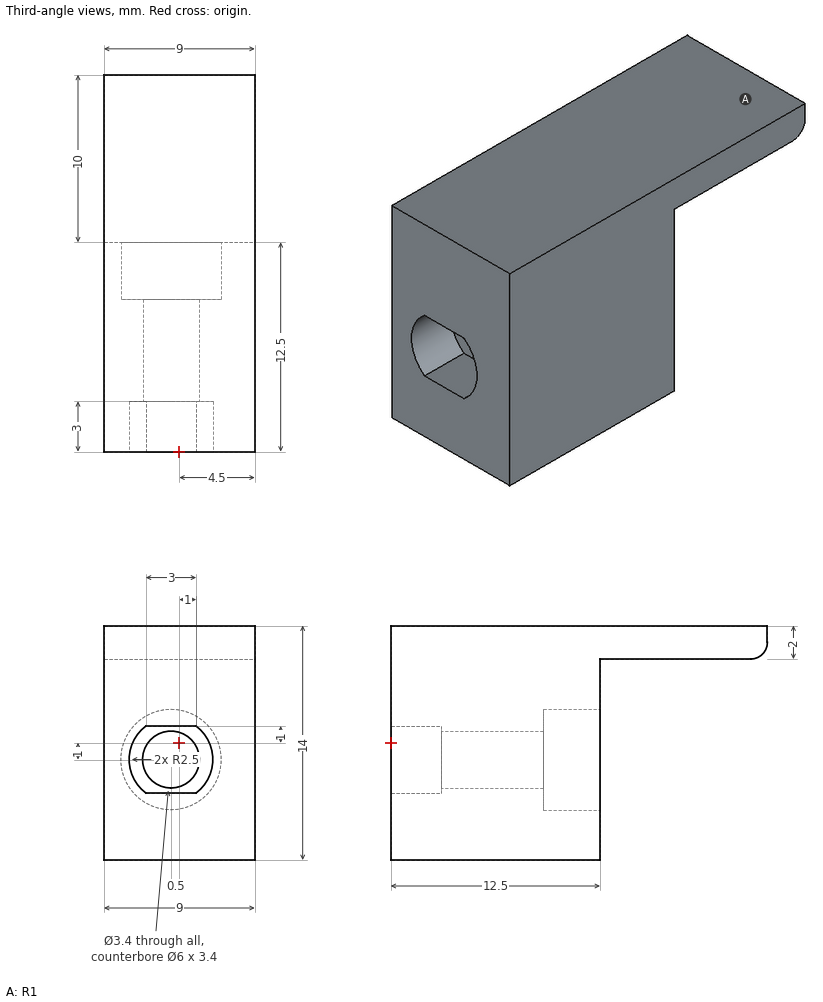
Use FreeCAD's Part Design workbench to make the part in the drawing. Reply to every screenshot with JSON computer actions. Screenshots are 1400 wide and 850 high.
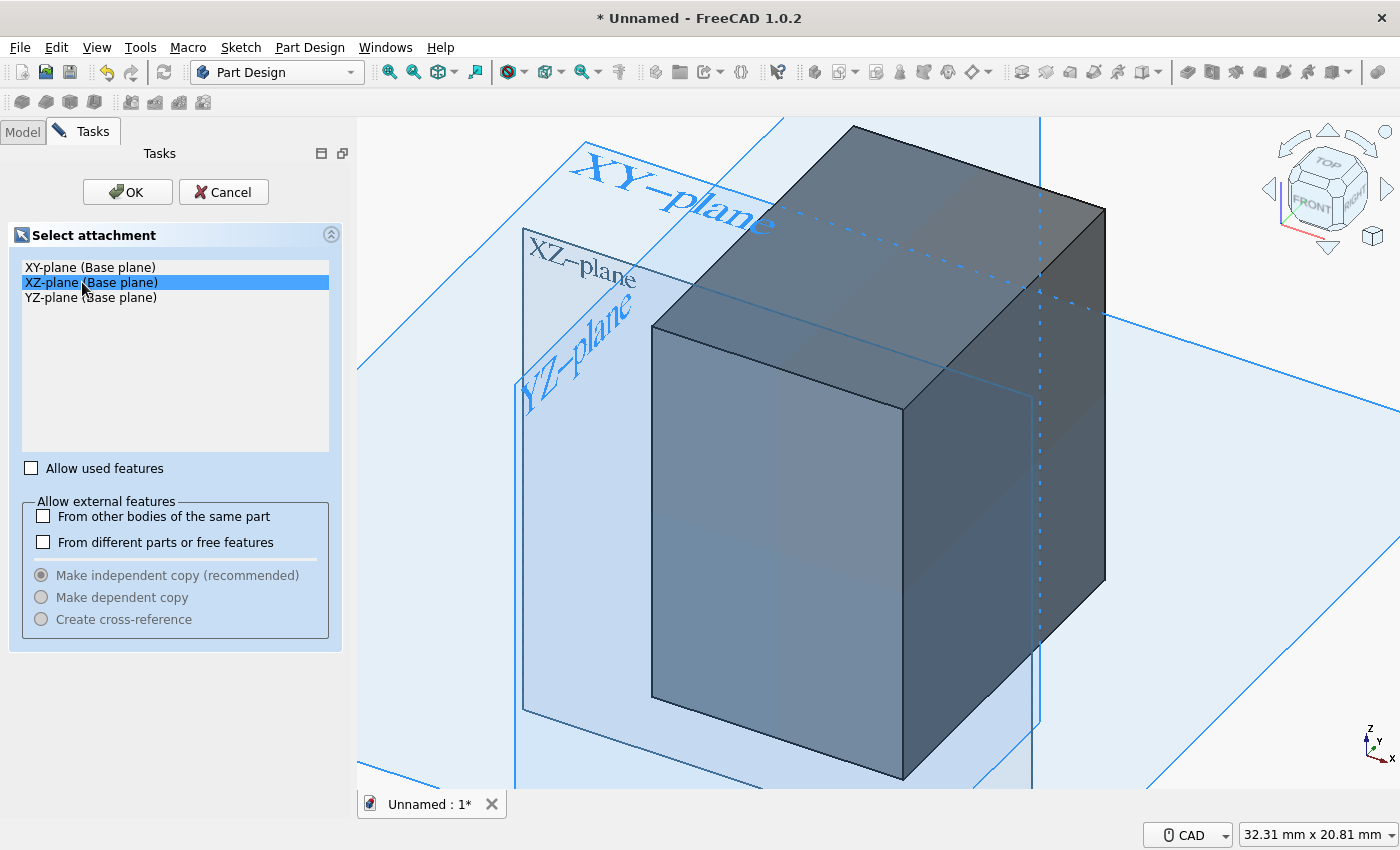
{"action": "left_click", "coordinate": [128, 192]}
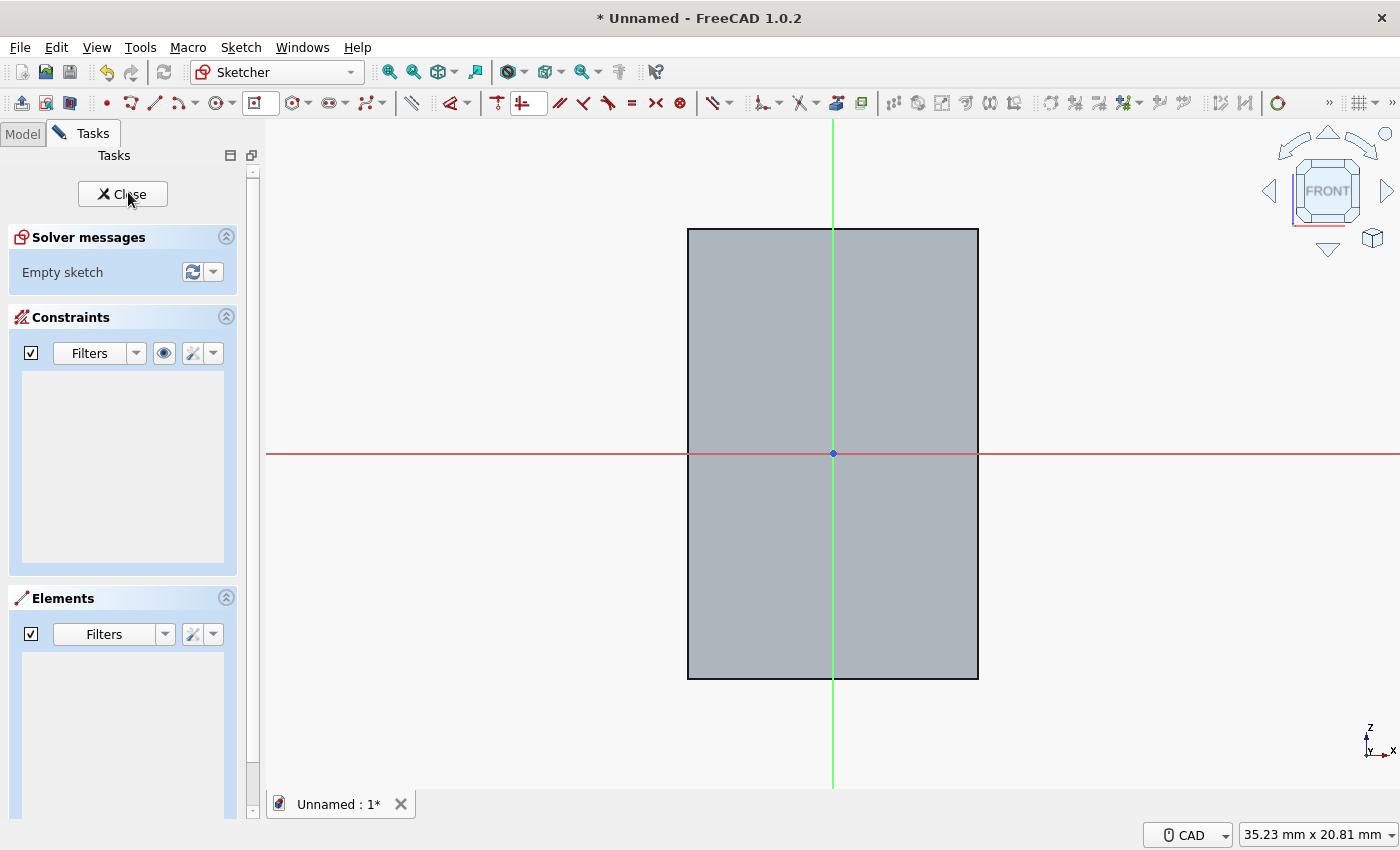
{"action": "scroll", "coordinate": [839, 500], "scroll_direction": "up", "scroll_amount": 6}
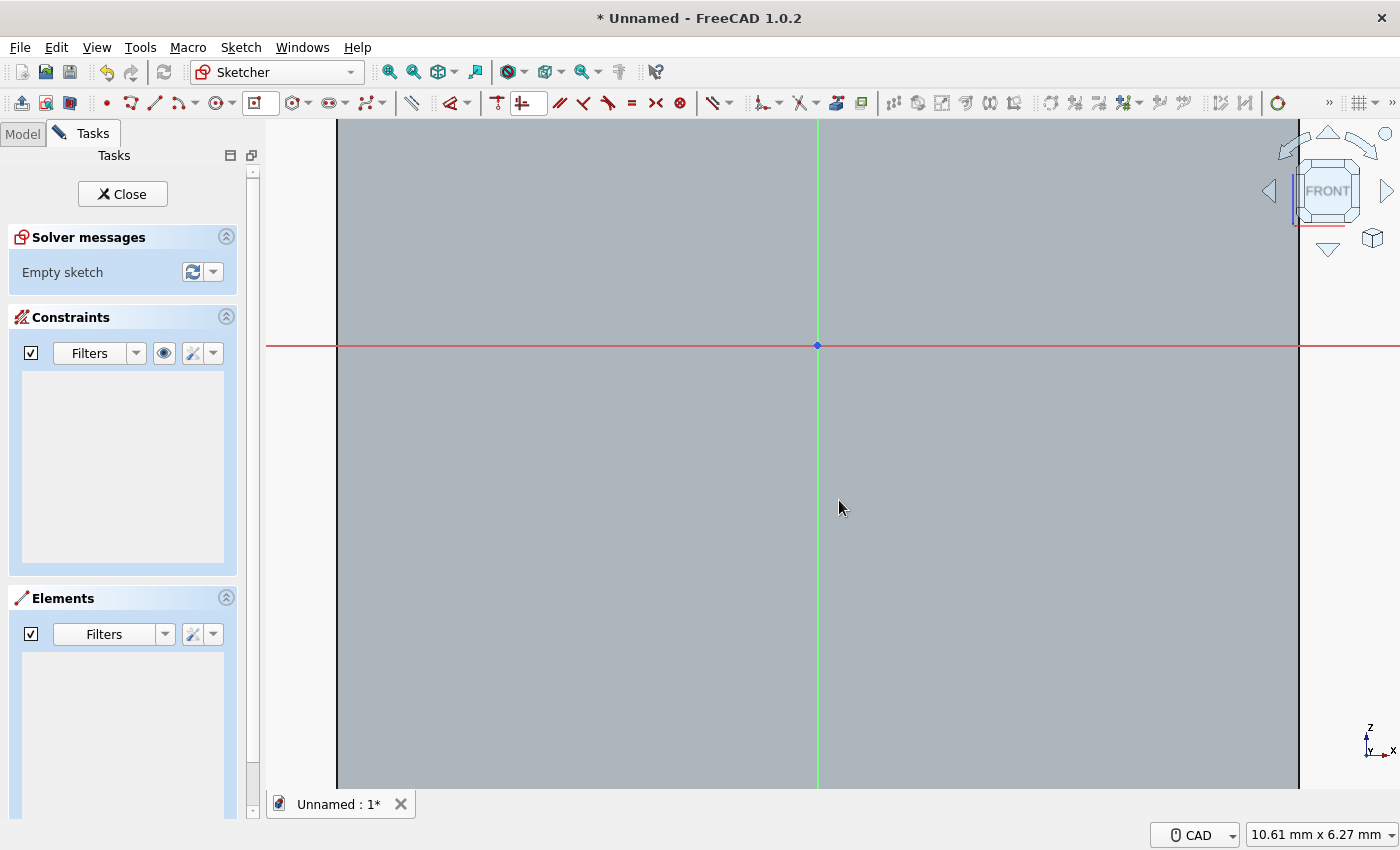
{"action": "key", "text": "g l"}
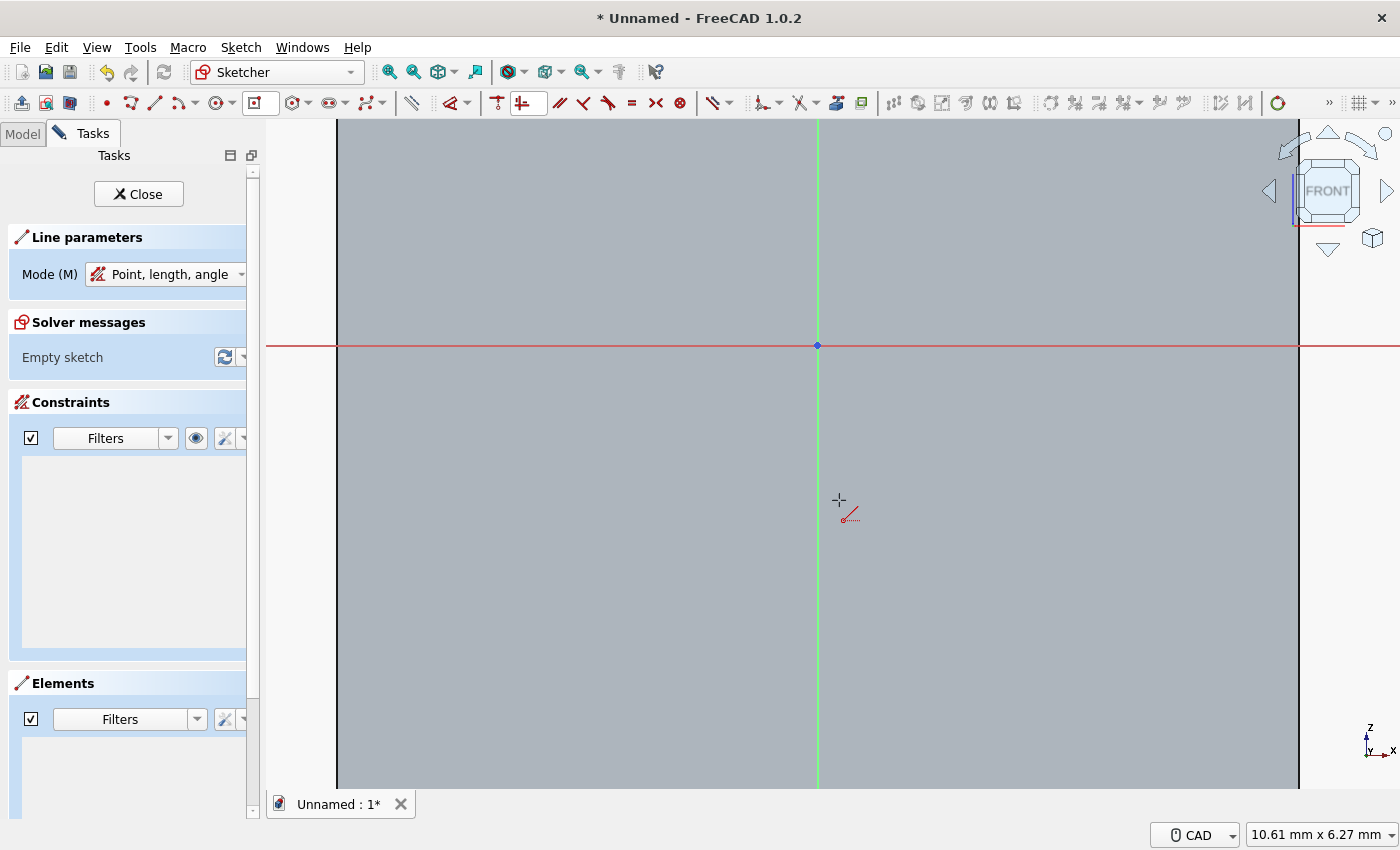
{"action": "left_click", "coordinate": [925, 239]}
{"action": "left_click", "coordinate": [604, 239]}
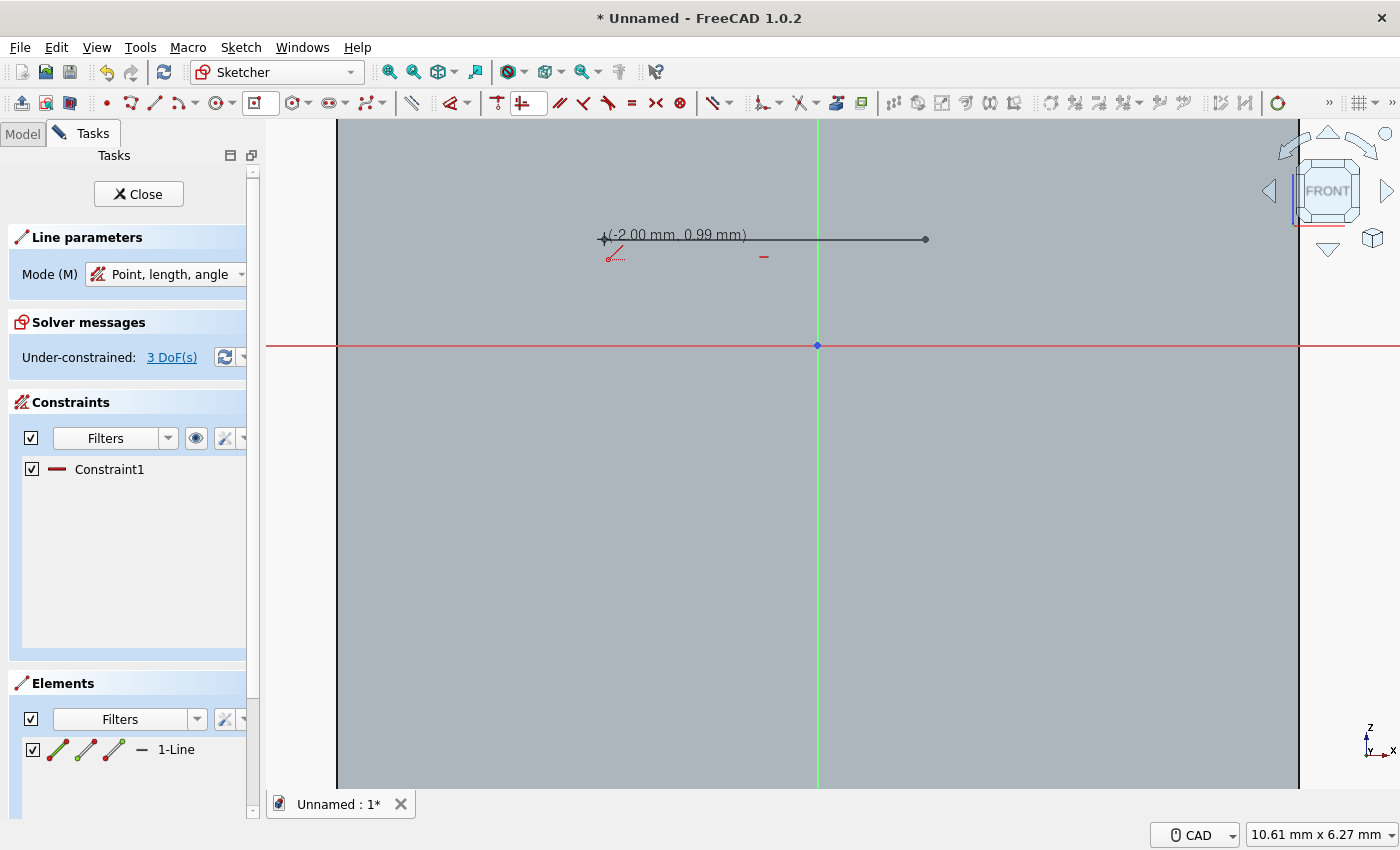
{"action": "left_click", "coordinate": [604, 667]}
{"action": "left_click", "coordinate": [925, 667]}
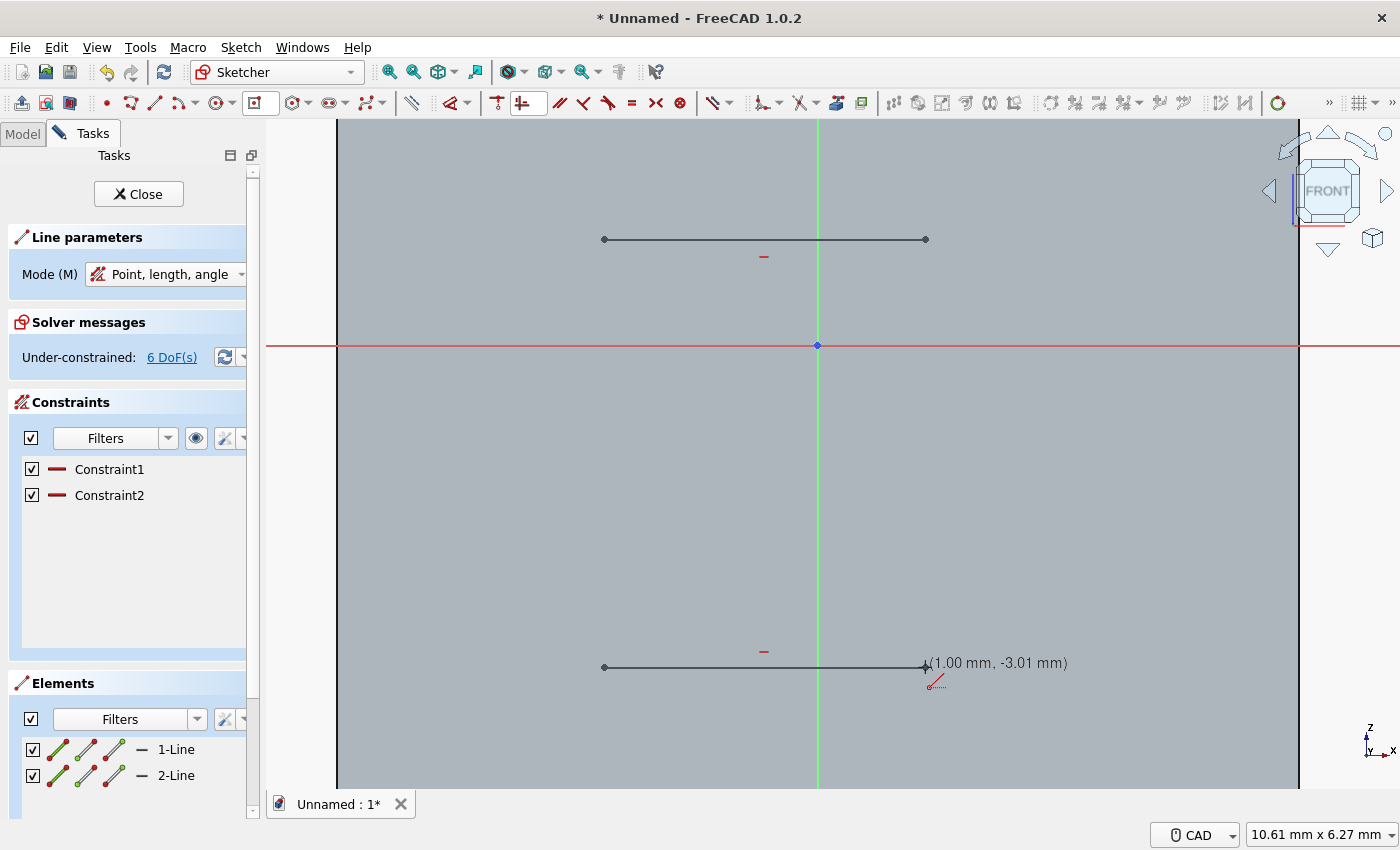
{"action": "key", "text": "g 3 a"}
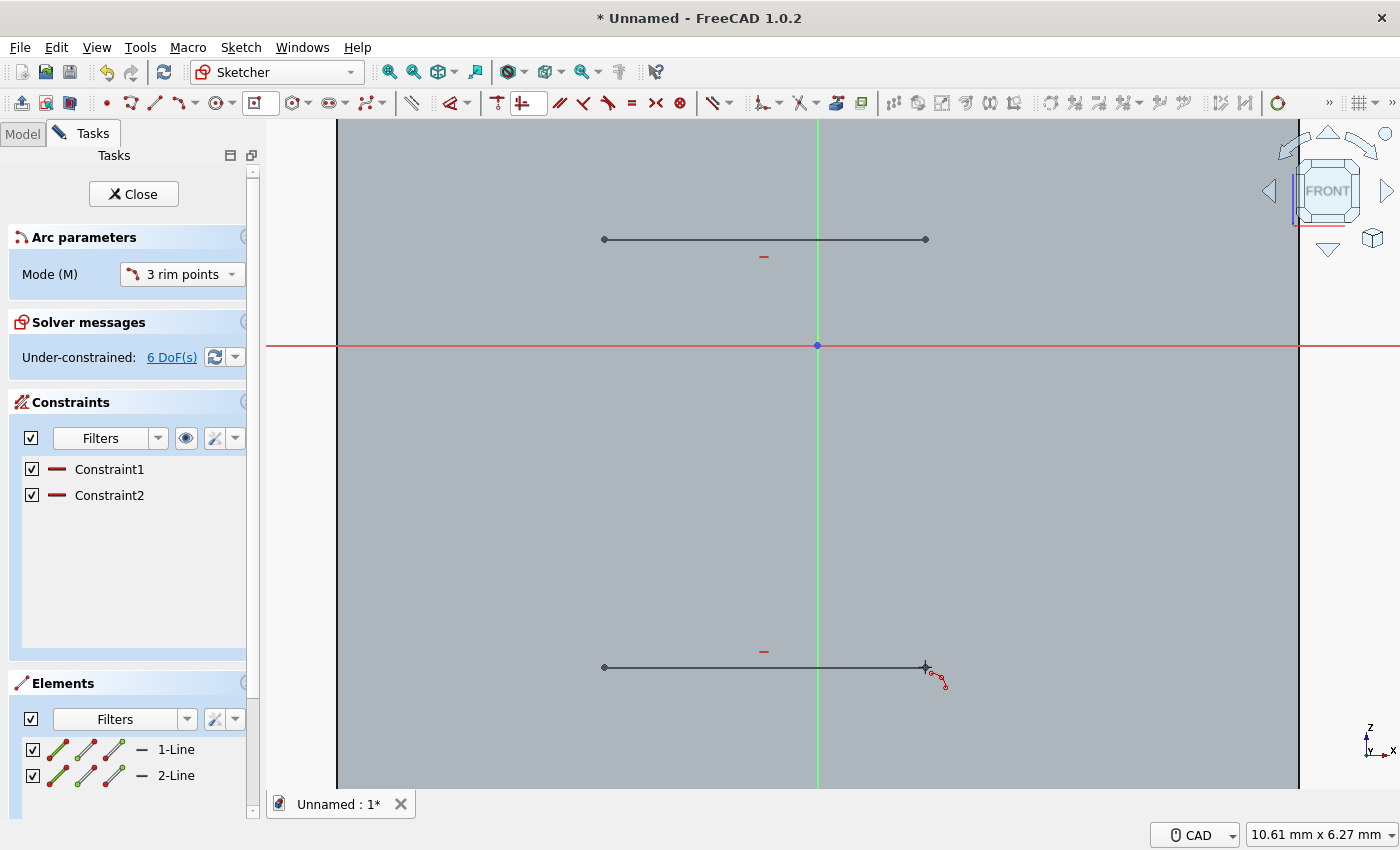
{"action": "left_click", "coordinate": [604, 240]}
{"action": "left_click", "coordinate": [604, 668]}
{"action": "left_click", "coordinate": [497, 453]}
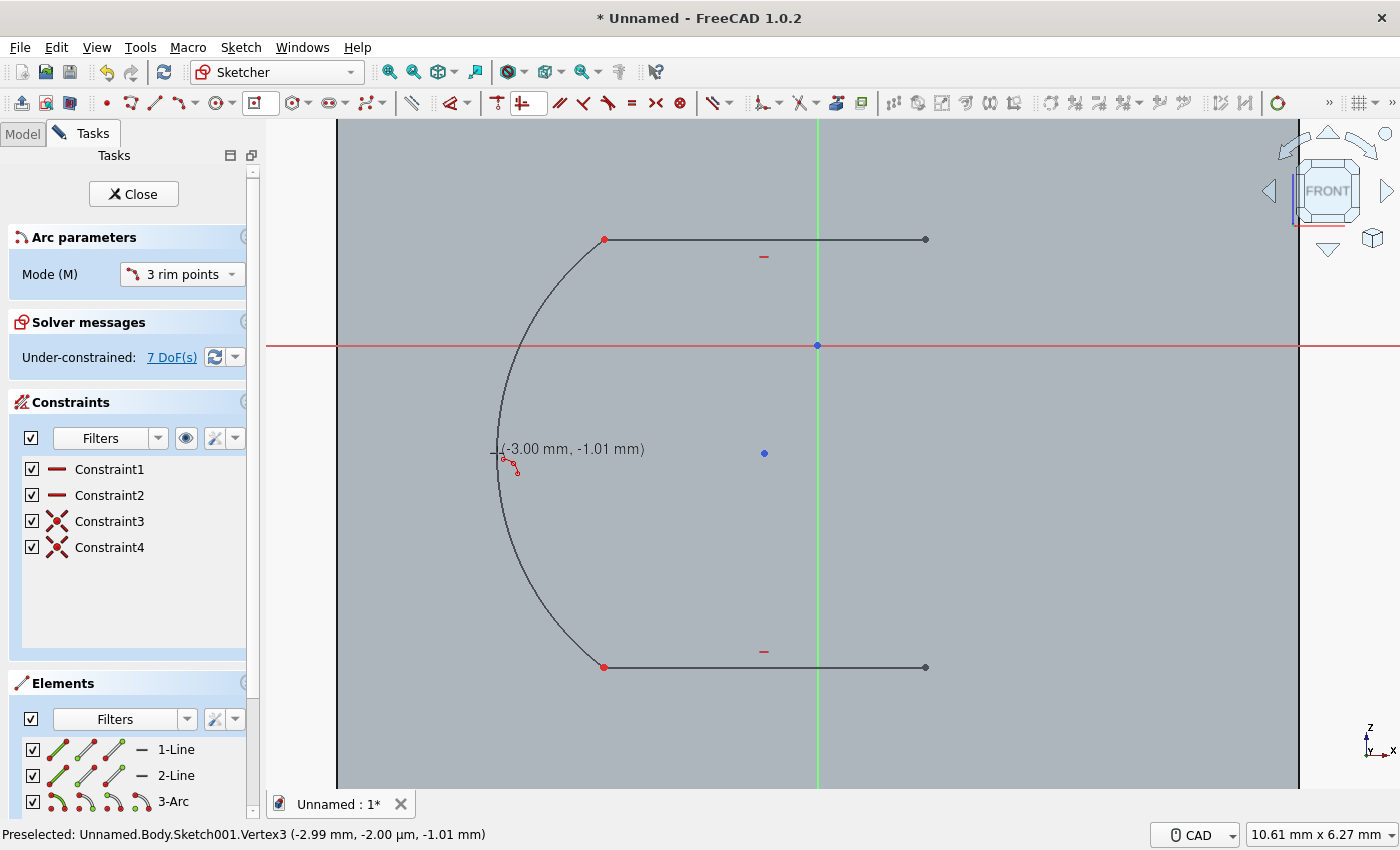
{"action": "left_click", "coordinate": [925, 668]}
{"action": "left_click", "coordinate": [925, 240]}
{"action": "left_click", "coordinate": [1032, 453]}
{"action": "key", "text": "Escape"}